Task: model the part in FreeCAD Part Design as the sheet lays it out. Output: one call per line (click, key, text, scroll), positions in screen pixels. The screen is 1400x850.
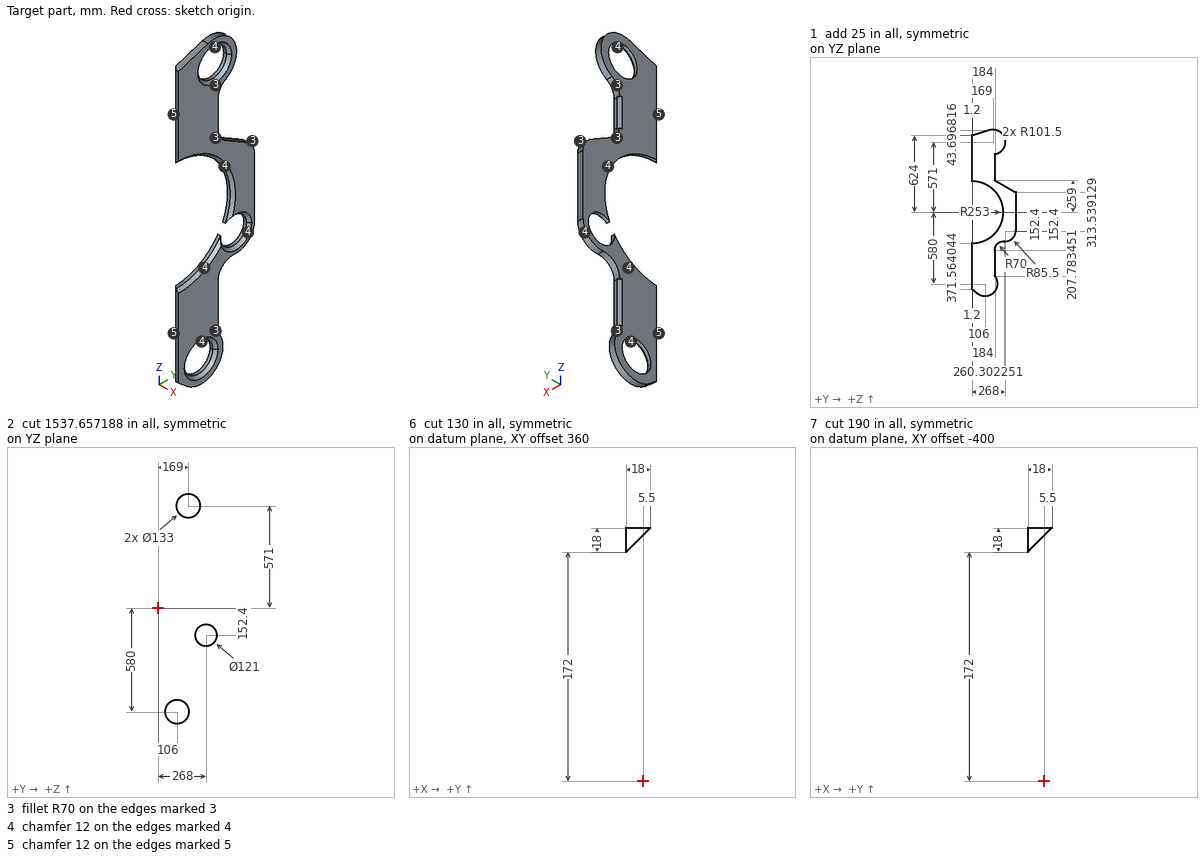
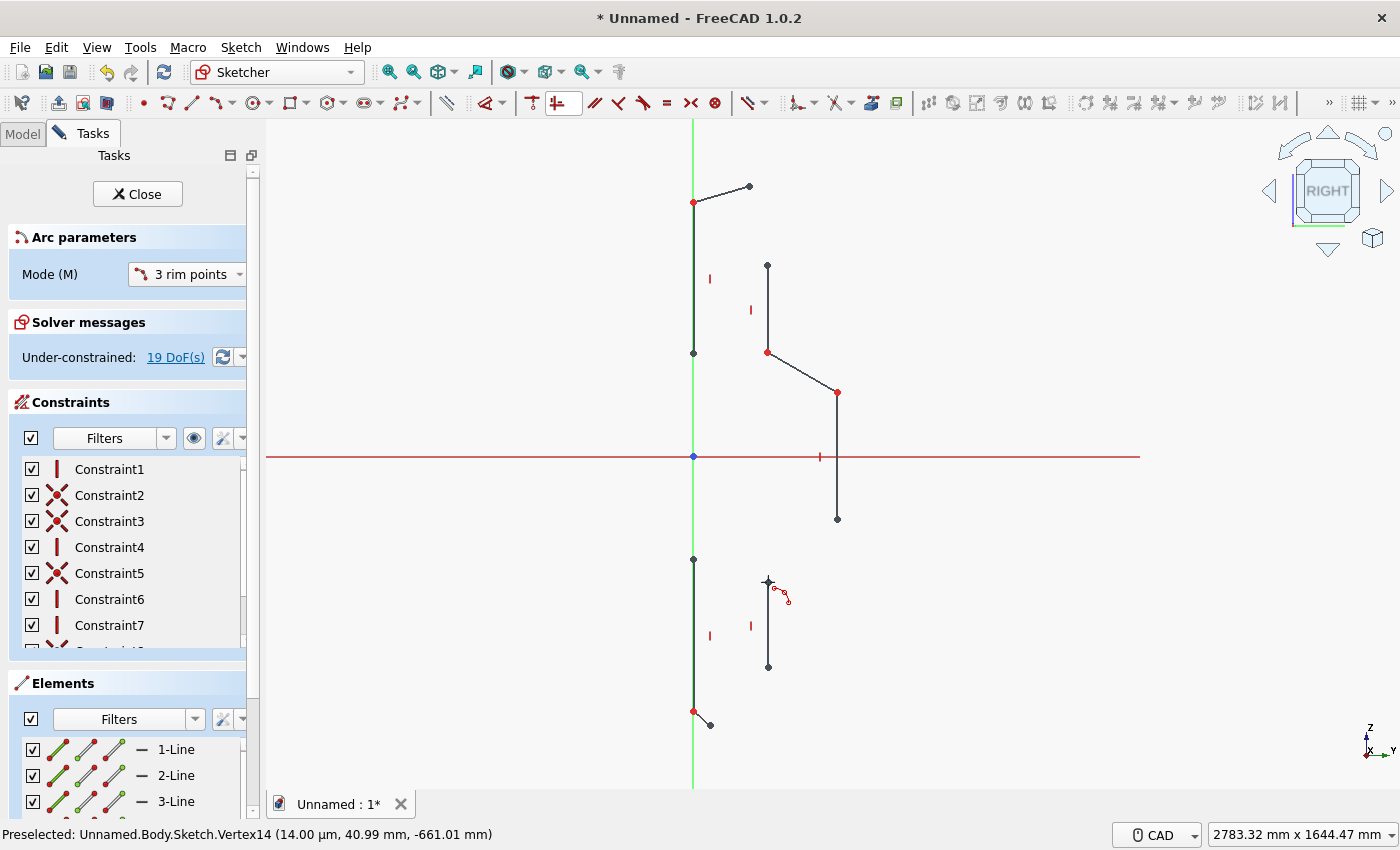
click(768, 266)
click(749, 186)
click(802, 215)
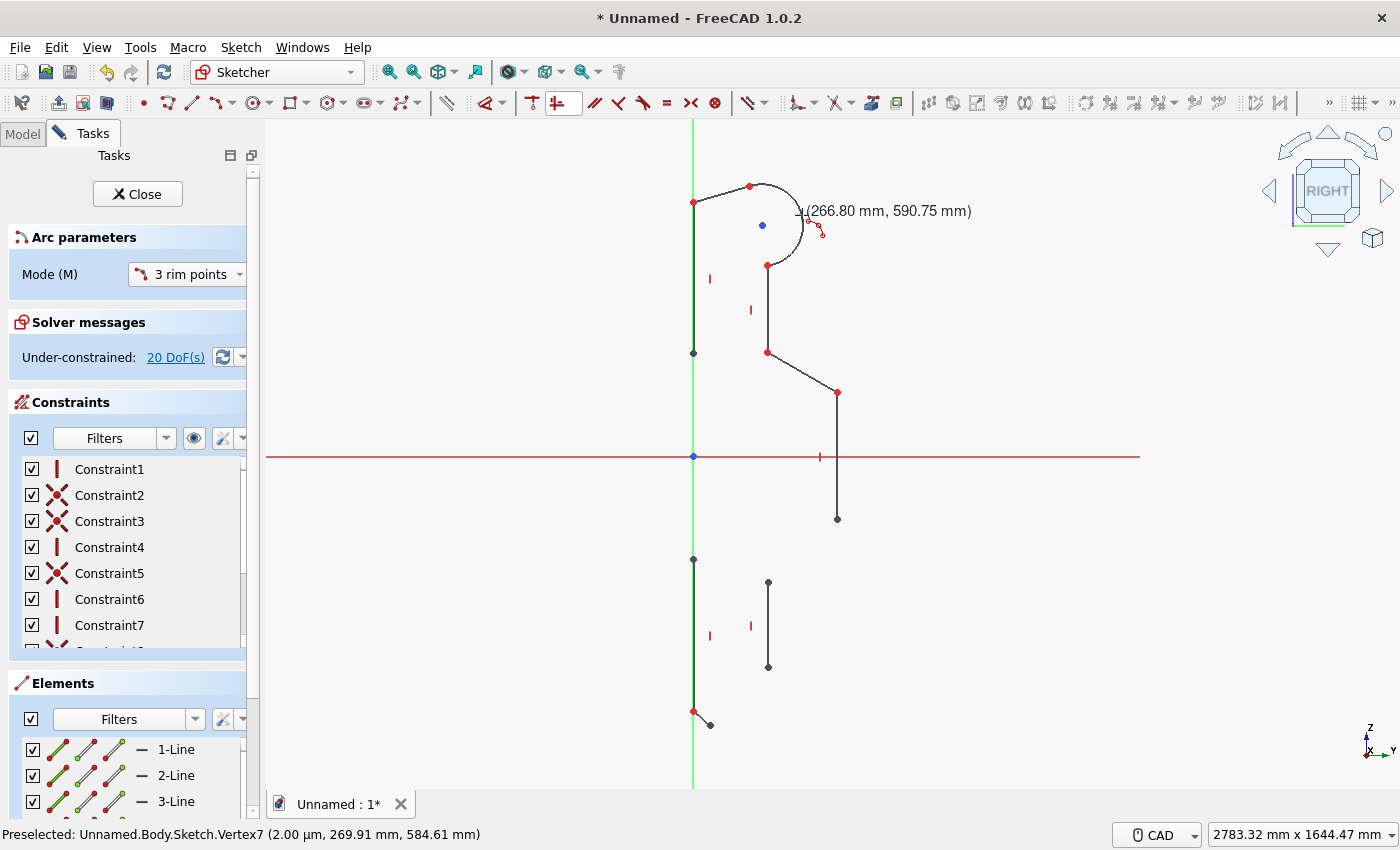
scroll(694, 354, up, 18)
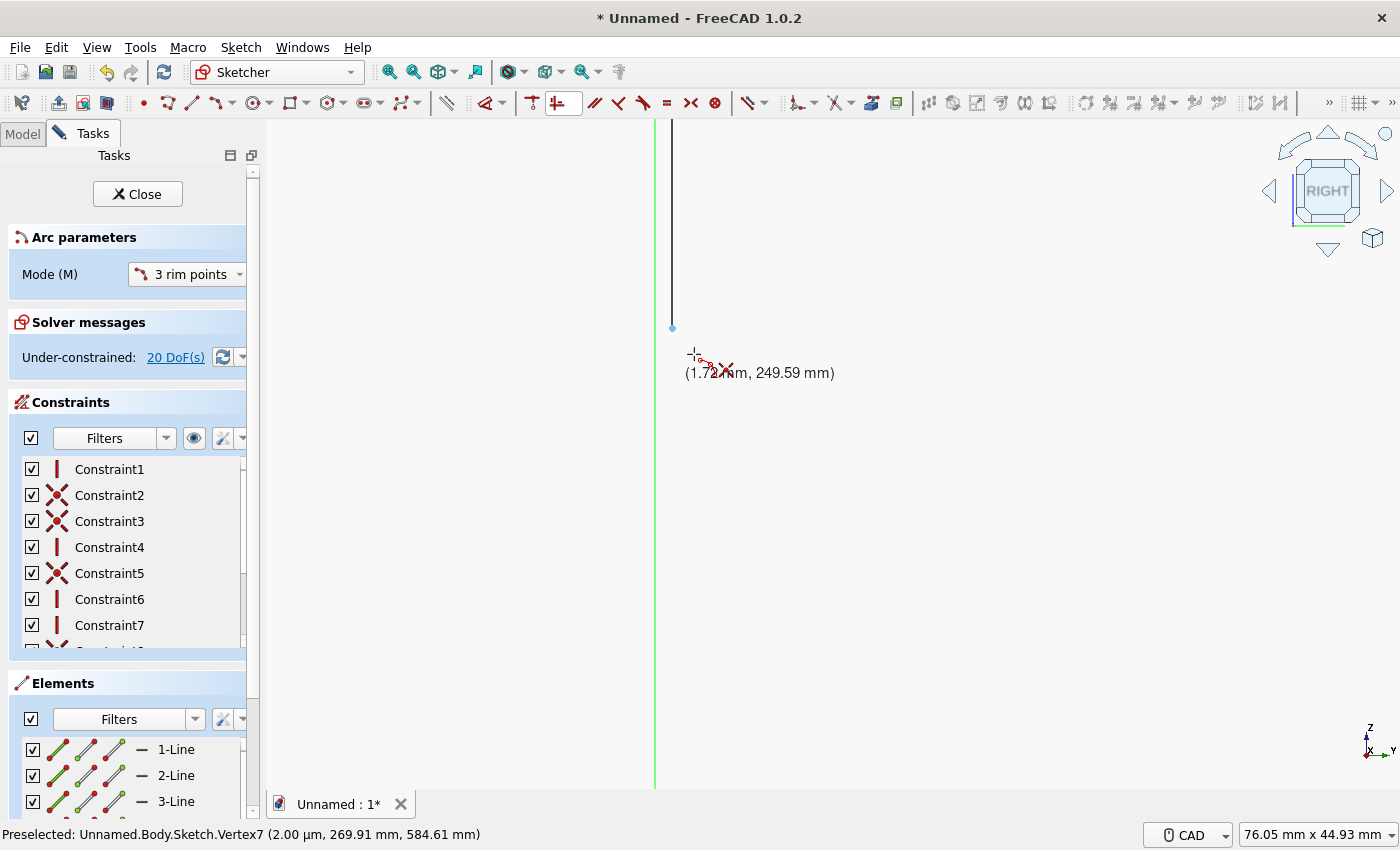
click(672, 328)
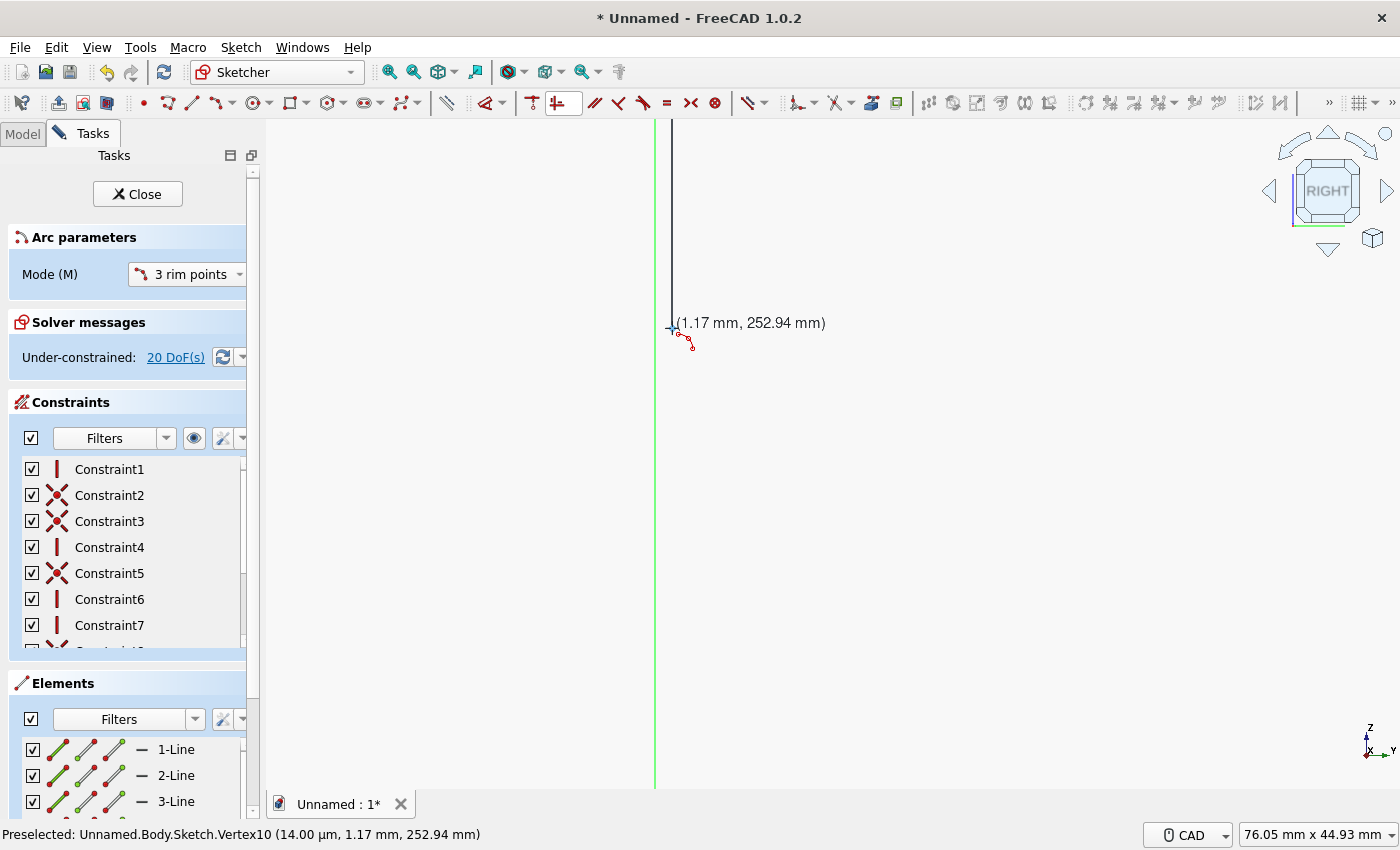
scroll(694, 354, down, 18)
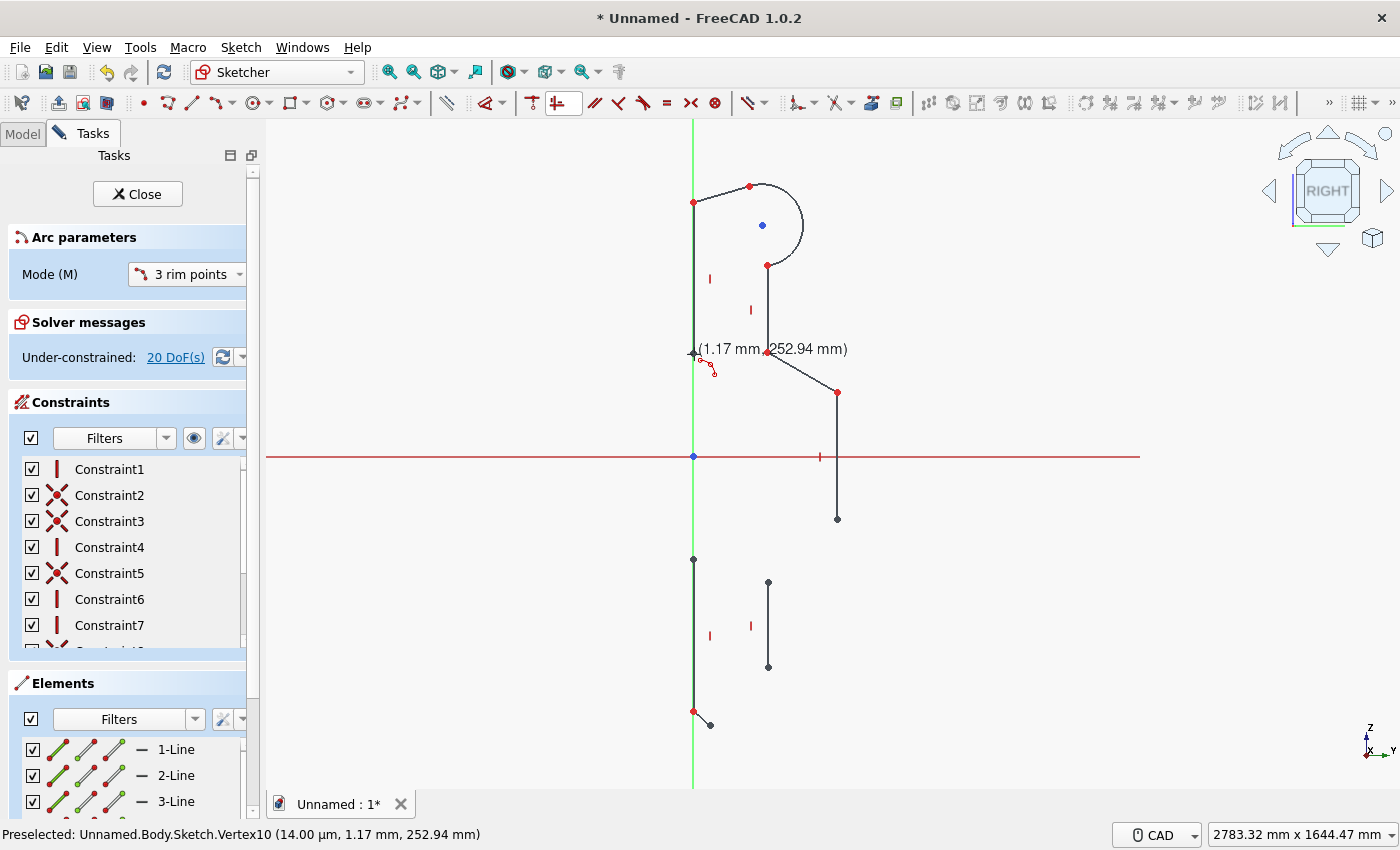
scroll(694, 560, up, 18)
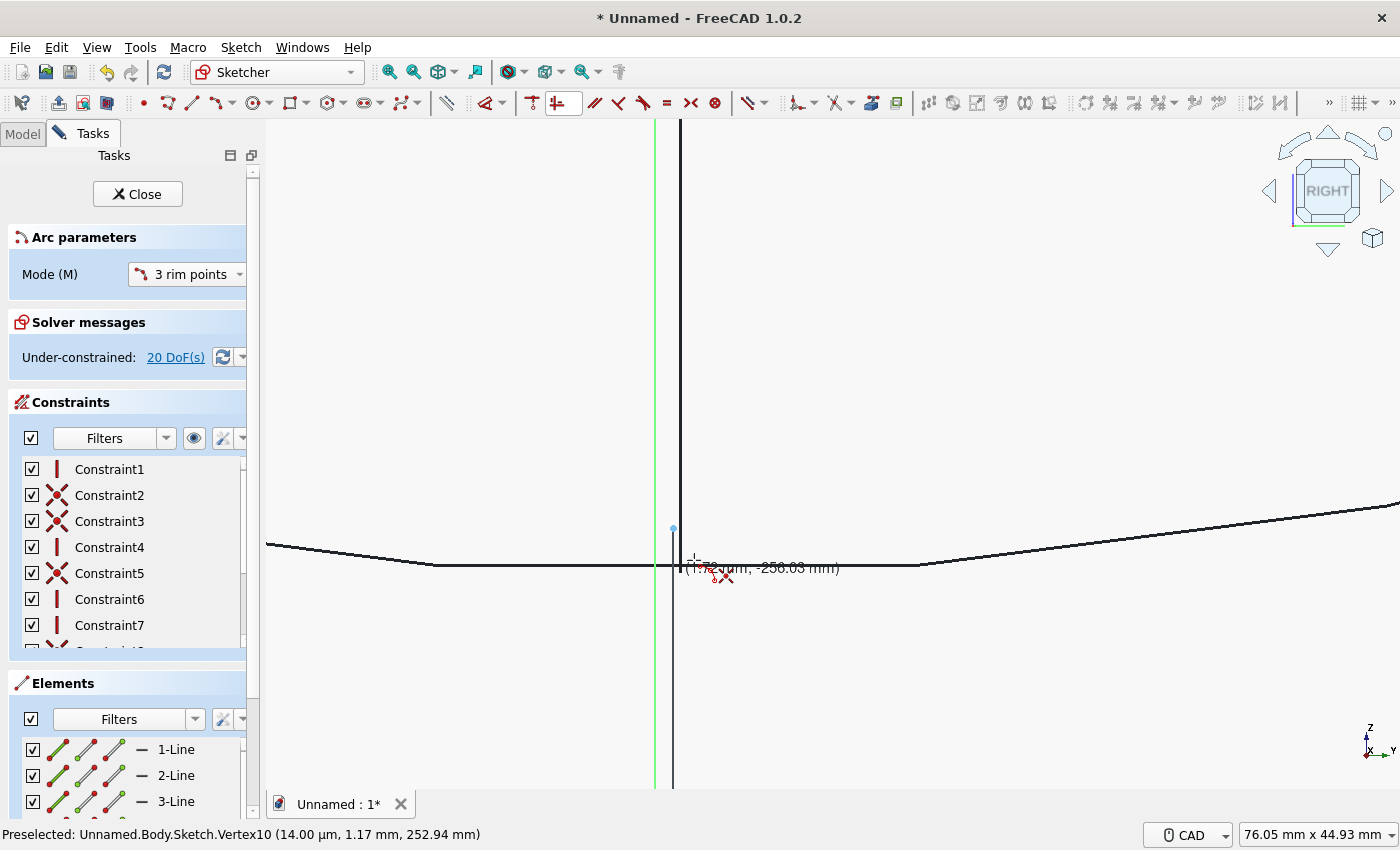
click(673, 529)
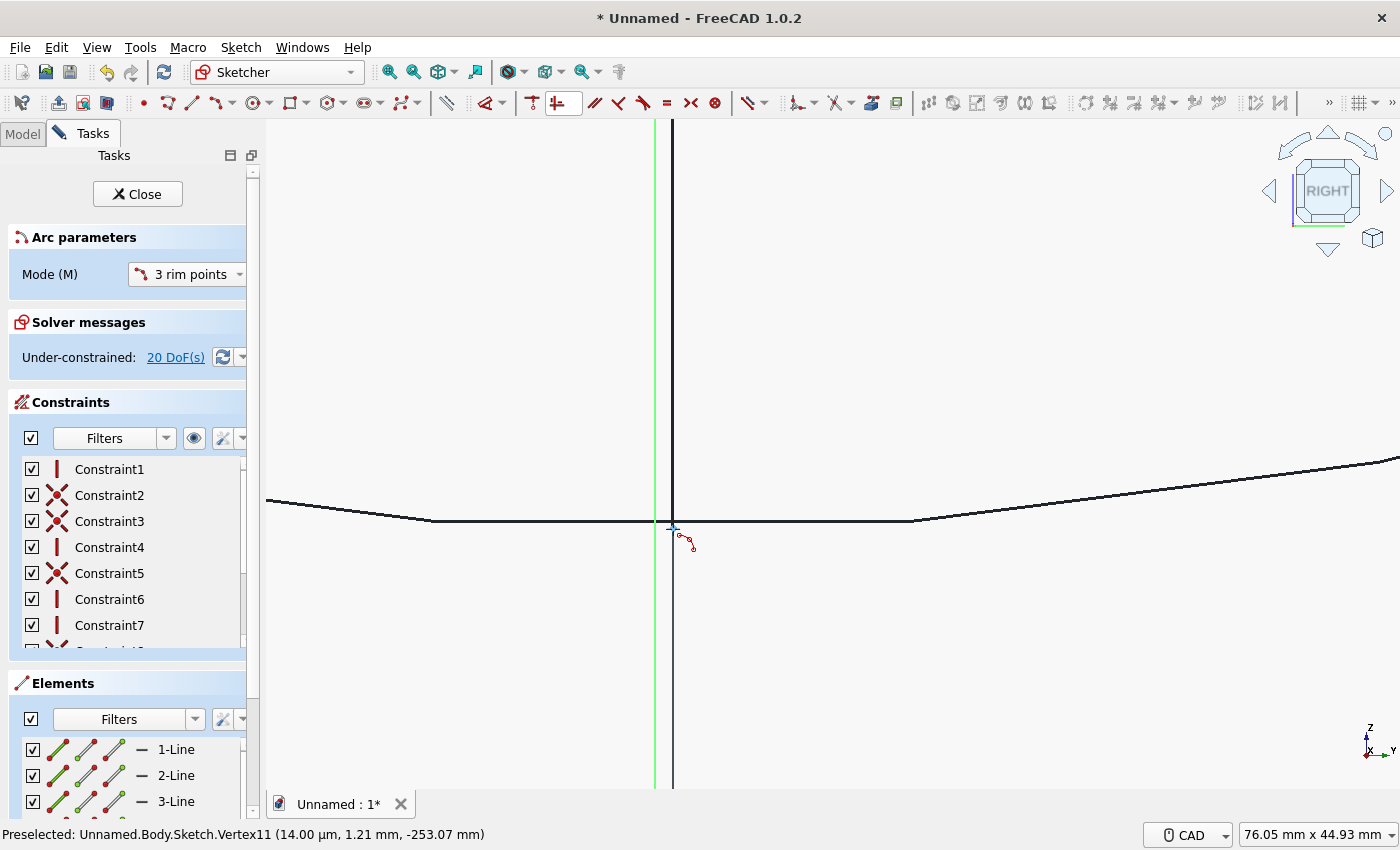
scroll(694, 560, down, 18)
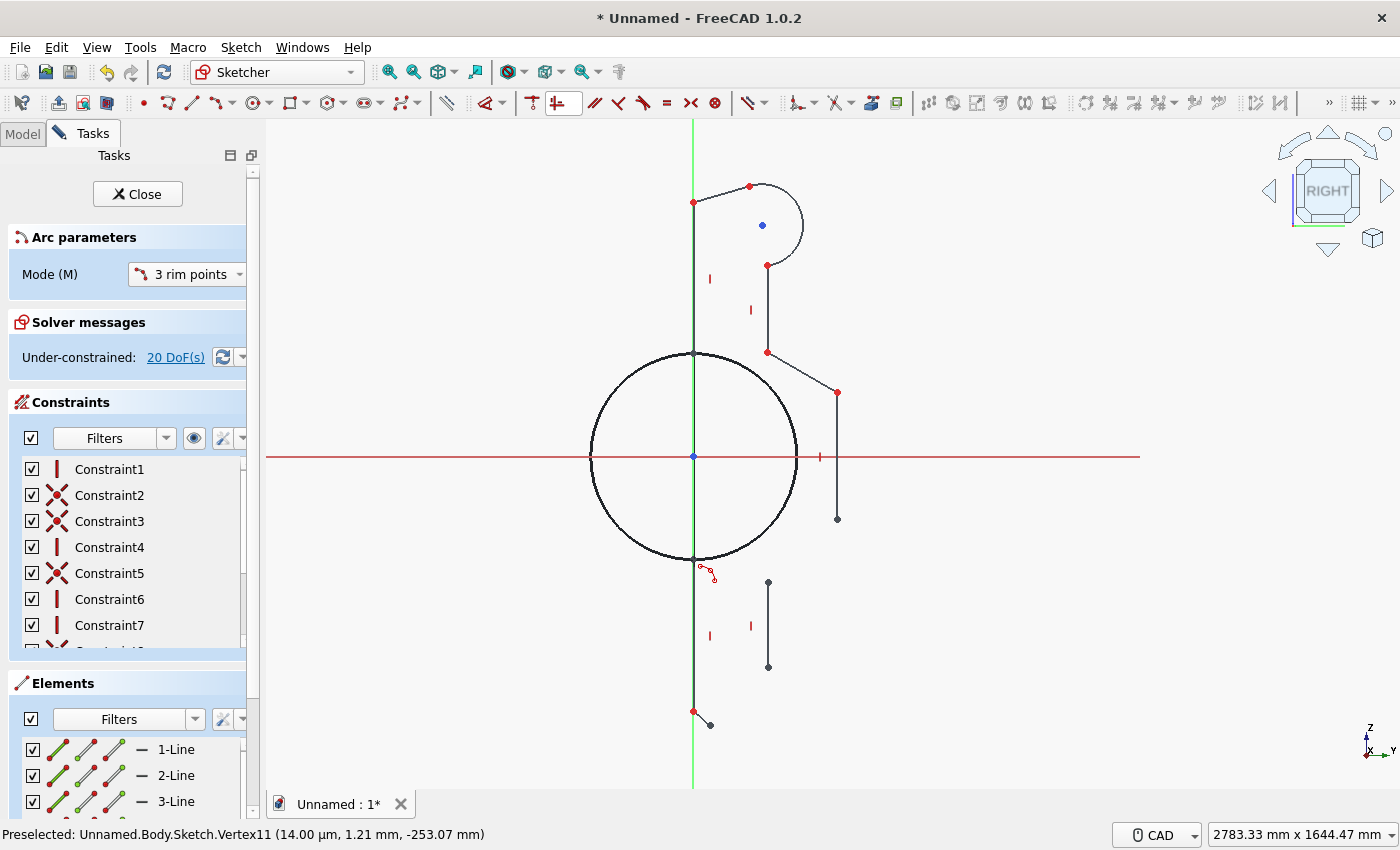
click(791, 488)